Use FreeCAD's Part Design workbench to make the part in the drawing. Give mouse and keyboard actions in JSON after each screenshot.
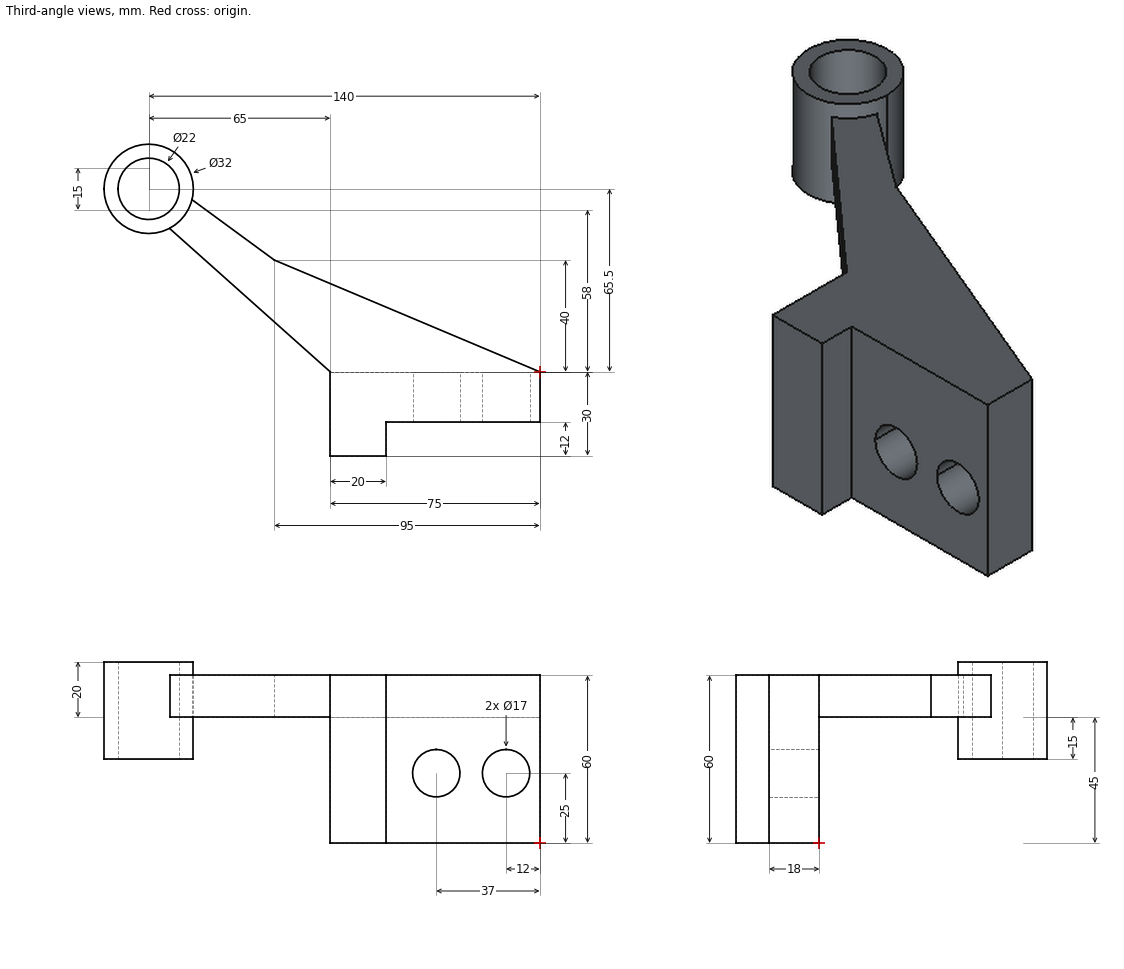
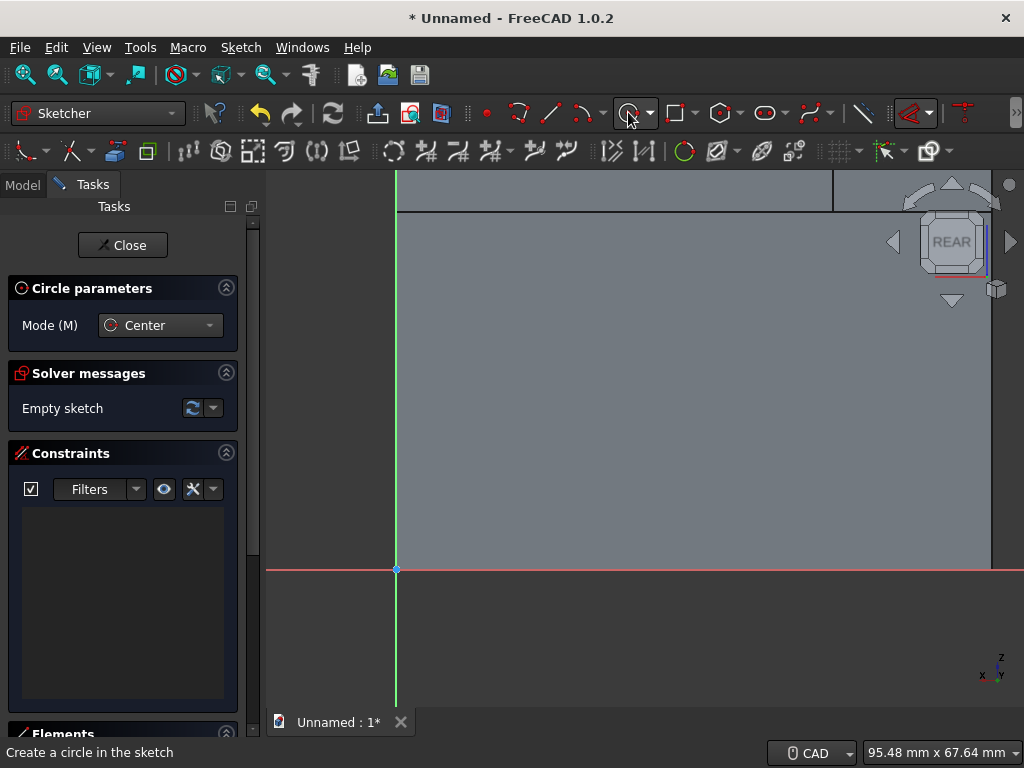
{"action": "left_click", "coordinate": [491, 371]}
{"action": "left_click", "coordinate": [539, 323]}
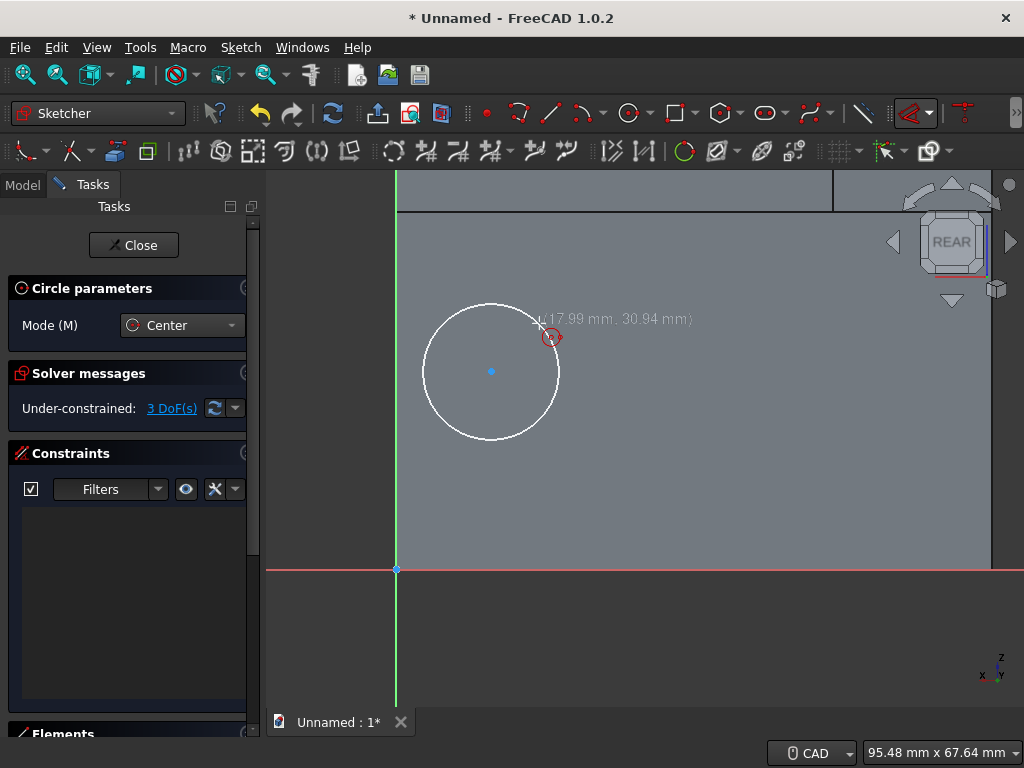
{"action": "left_click", "coordinate": [690, 371]}
{"action": "left_click", "coordinate": [738, 323]}
{"action": "key", "text": "Escape"}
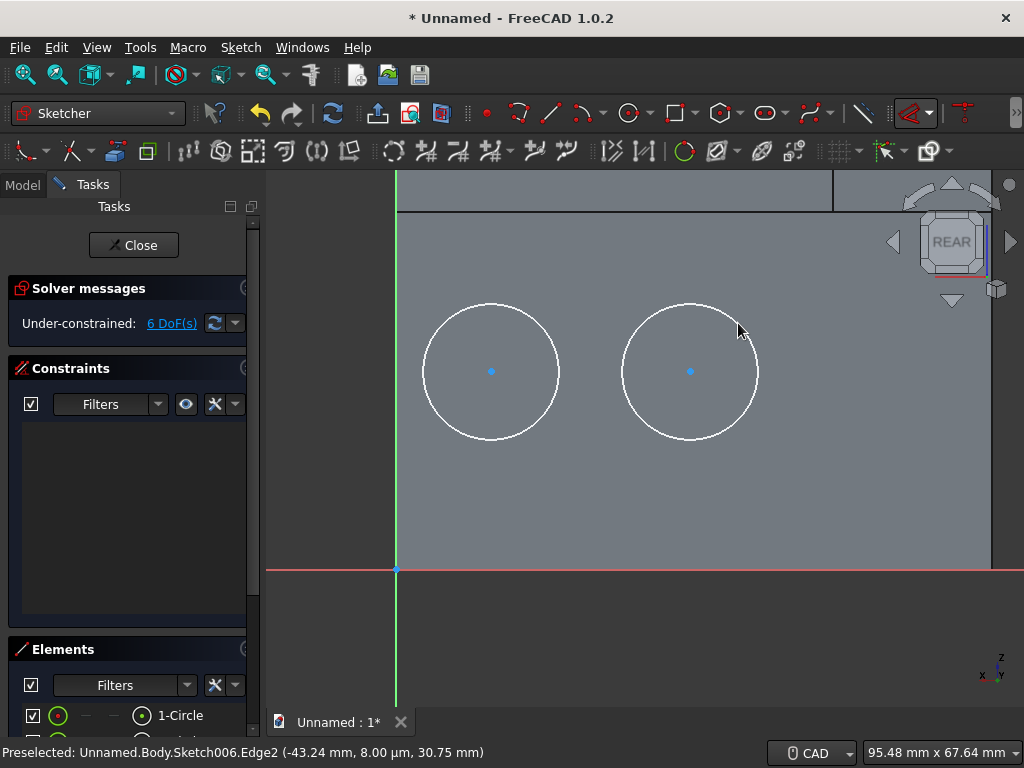
{"action": "left_click", "coordinate": [539, 324]}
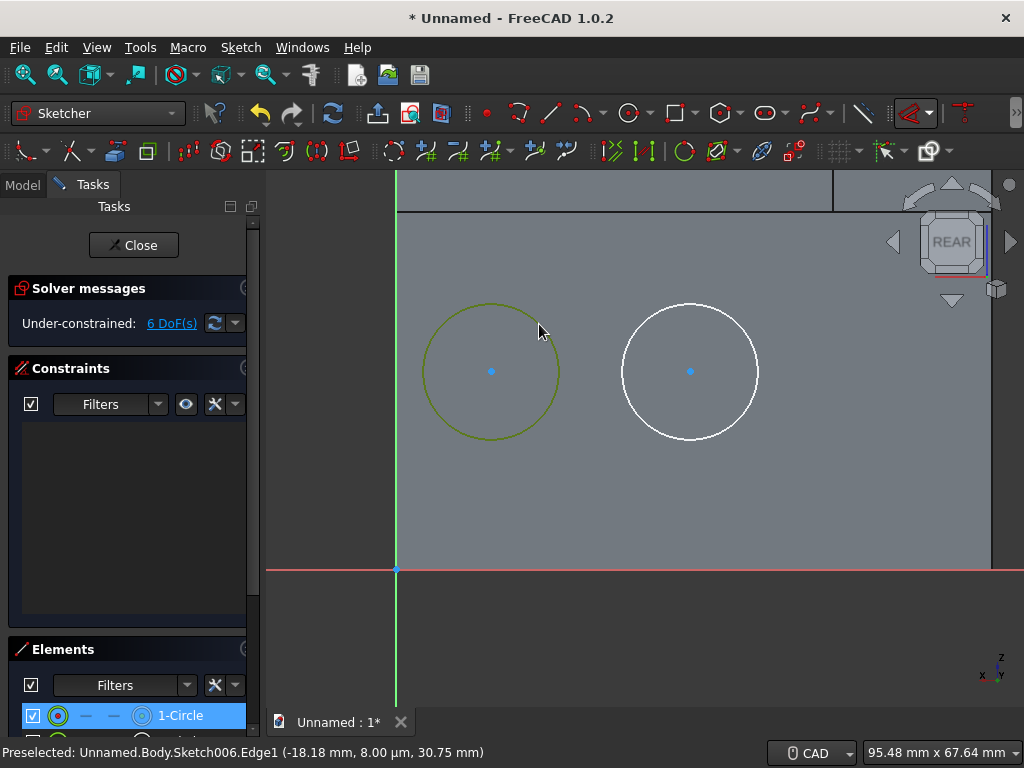
{"action": "left_click", "coordinate": [738, 324]}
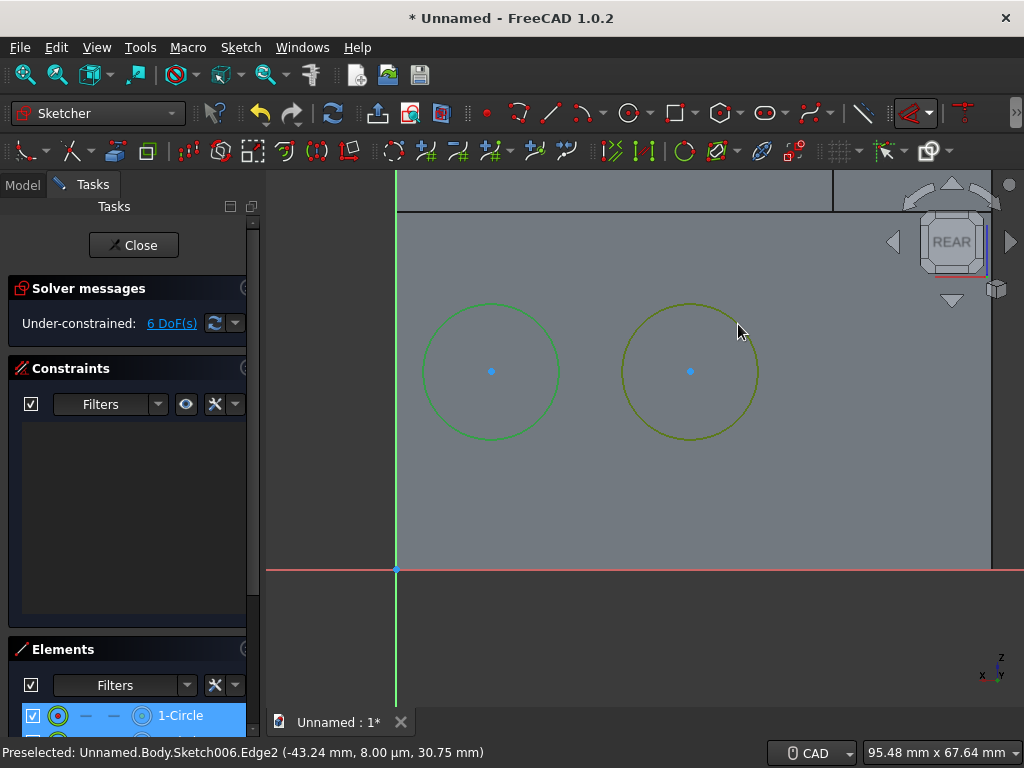
{"action": "key", "text": "e"}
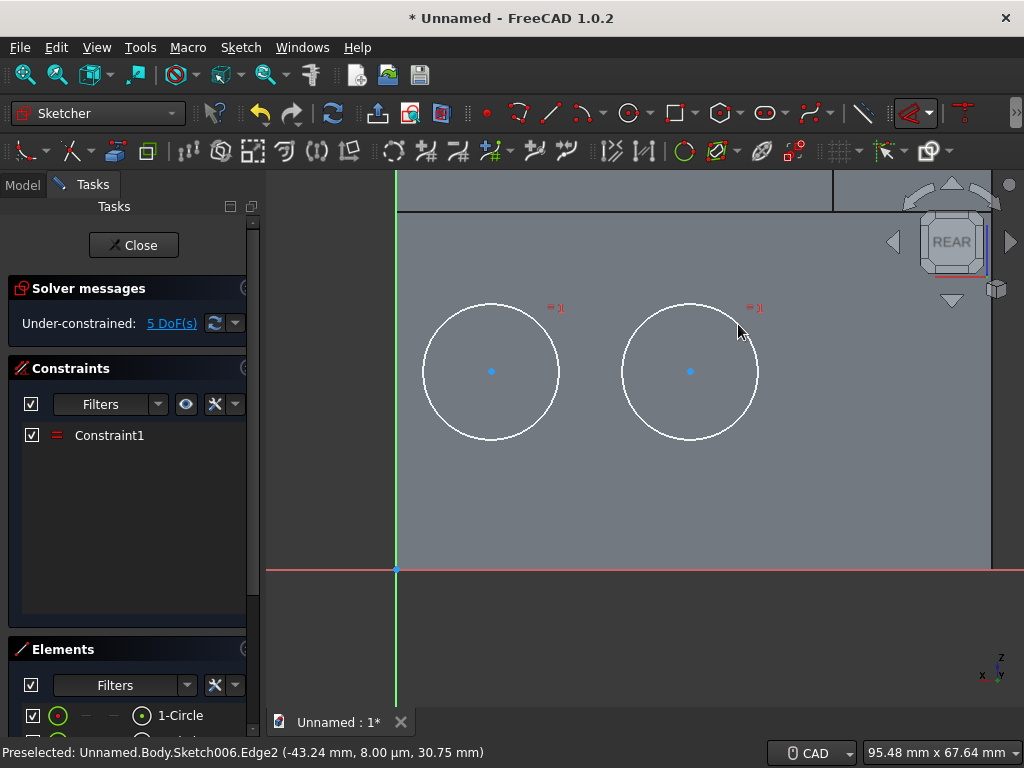
{"action": "left_click", "coordinate": [539, 324]}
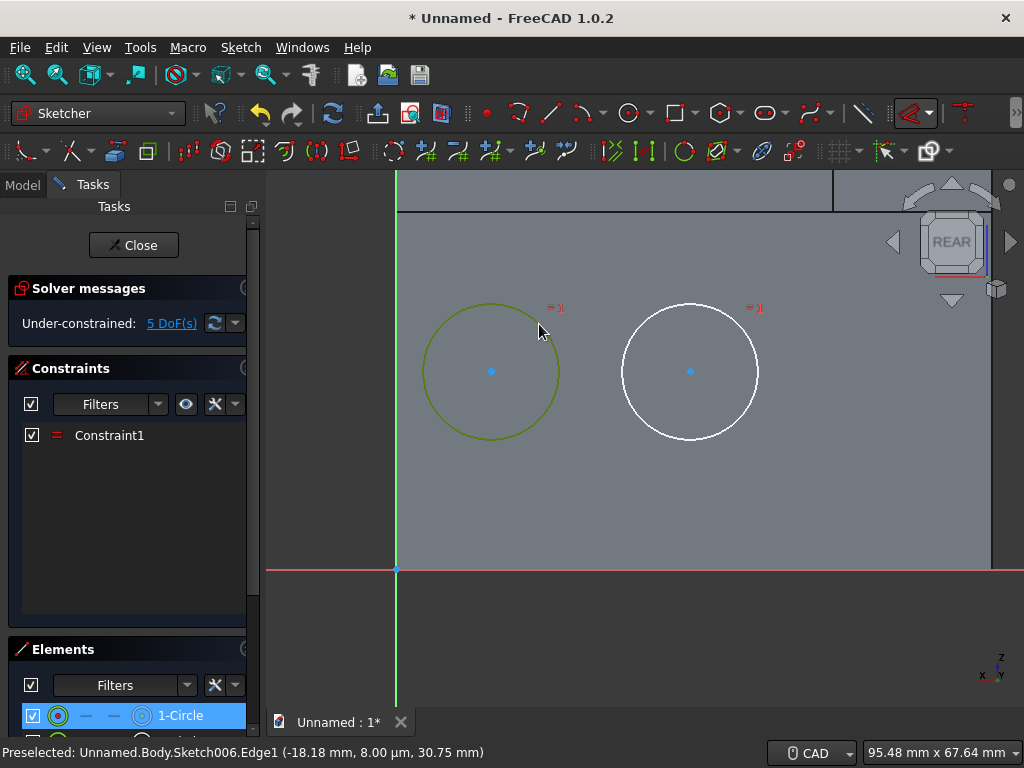
{"action": "key", "text": "k o"}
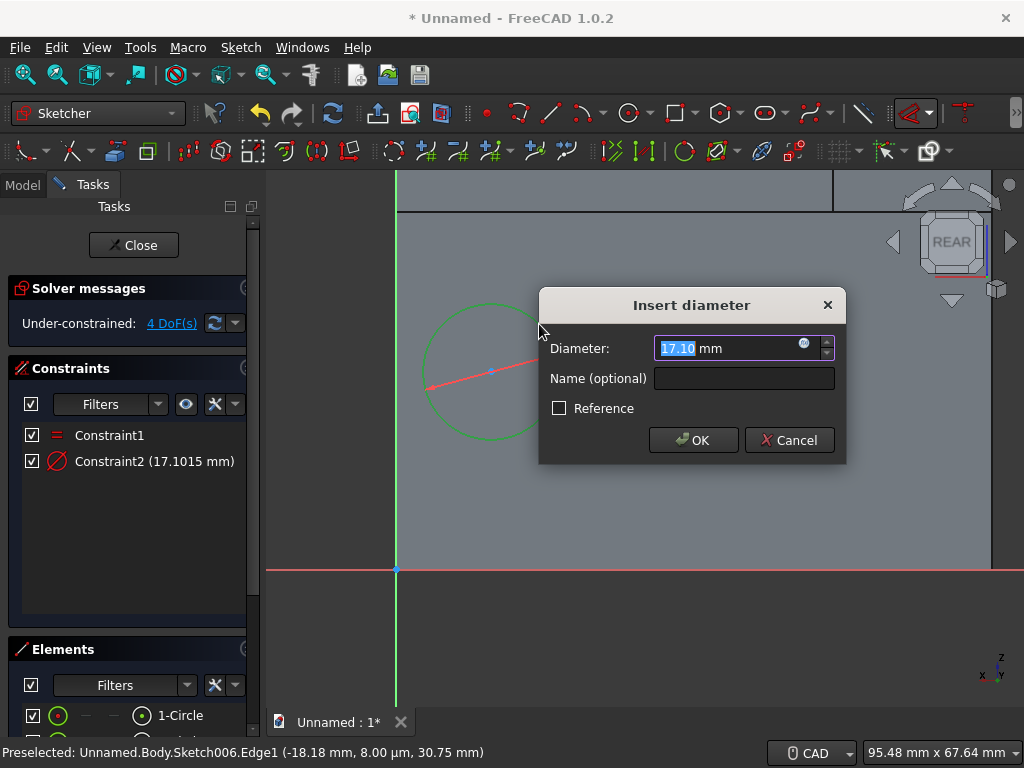
{"action": "type", "text": "17"}
{"action": "key", "text": "Return"}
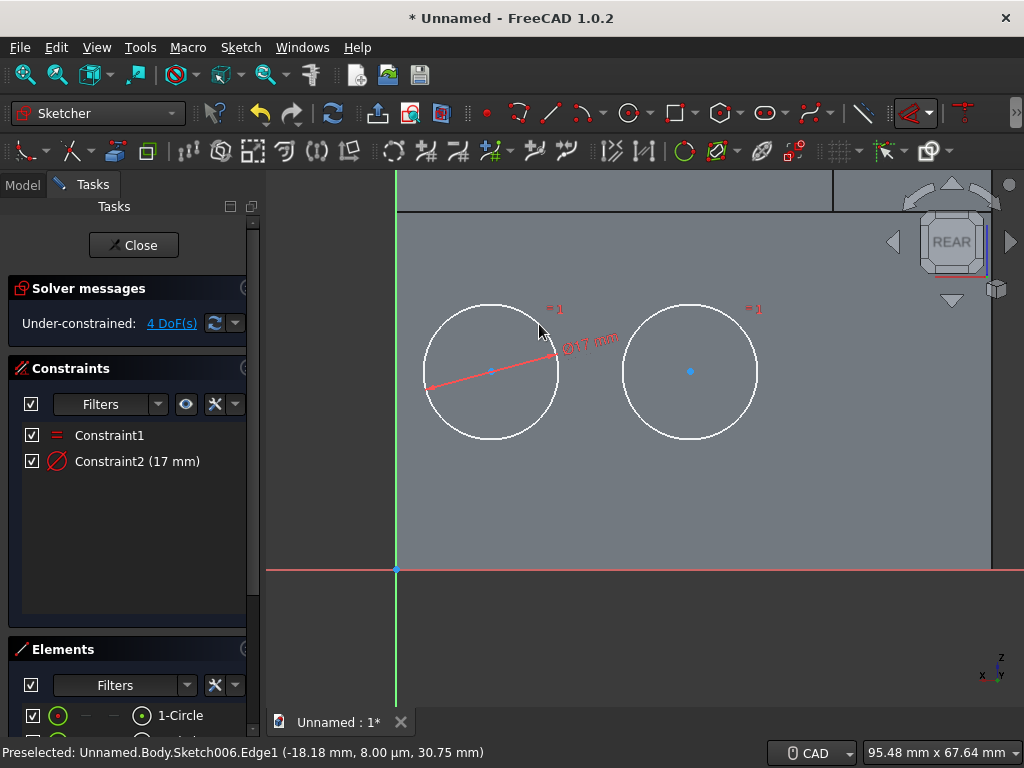
{"action": "left_click", "coordinate": [491, 372]}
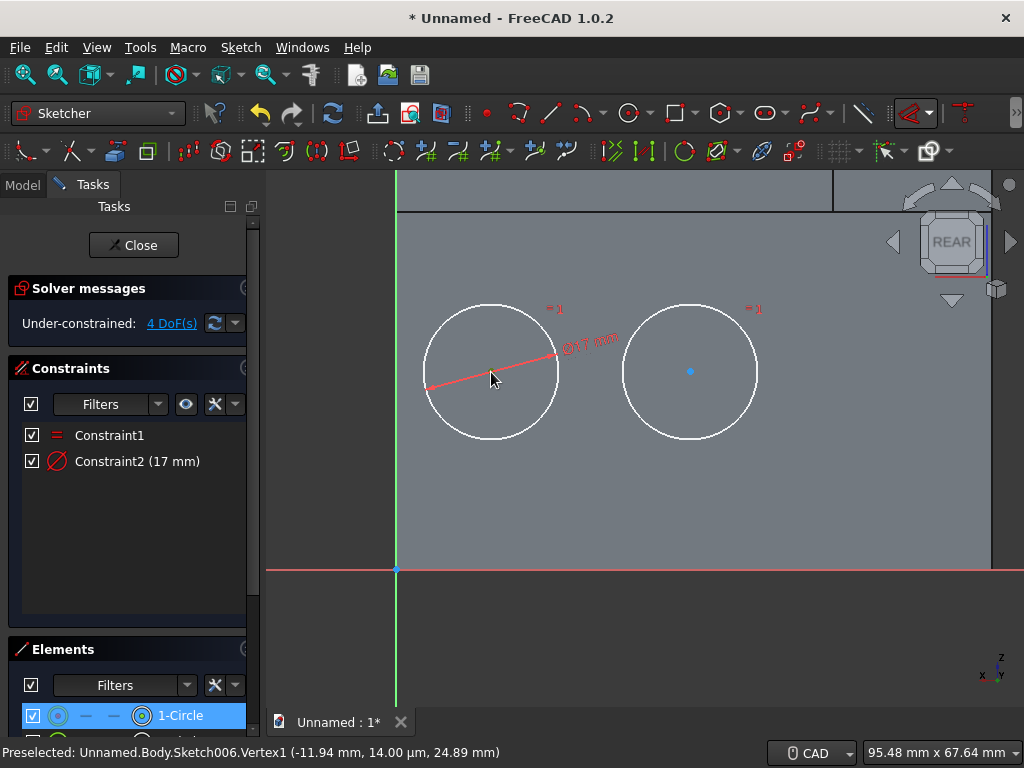
{"action": "key", "text": "l"}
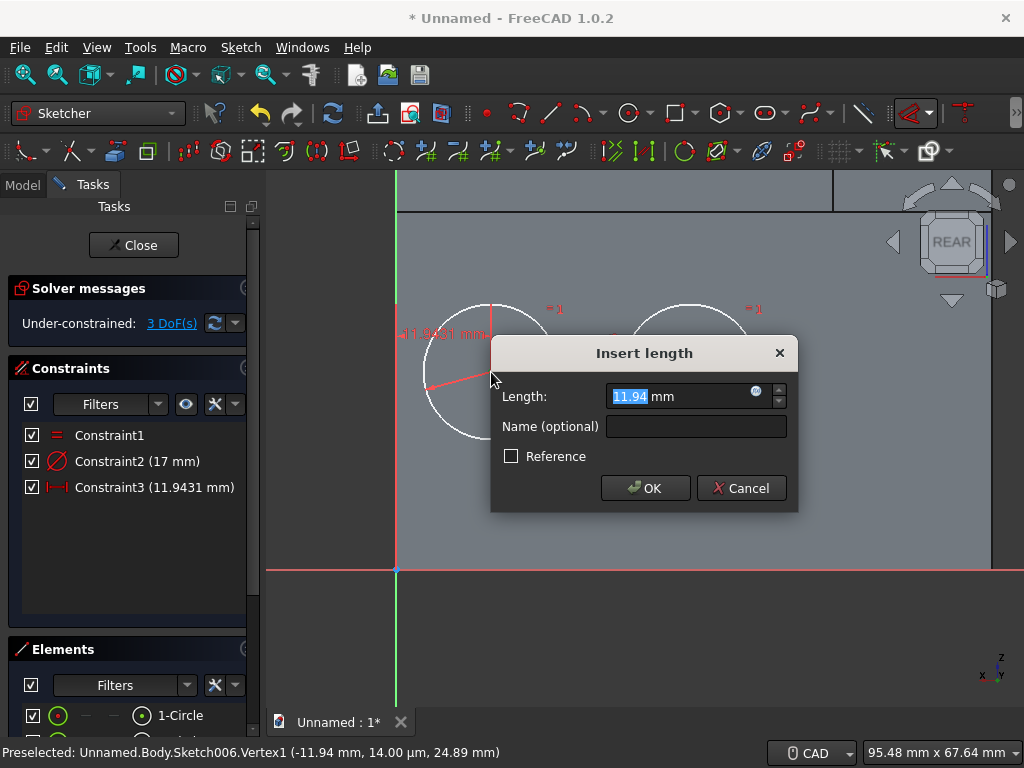
{"action": "type", "text": "12"}
{"action": "key", "text": "Return"}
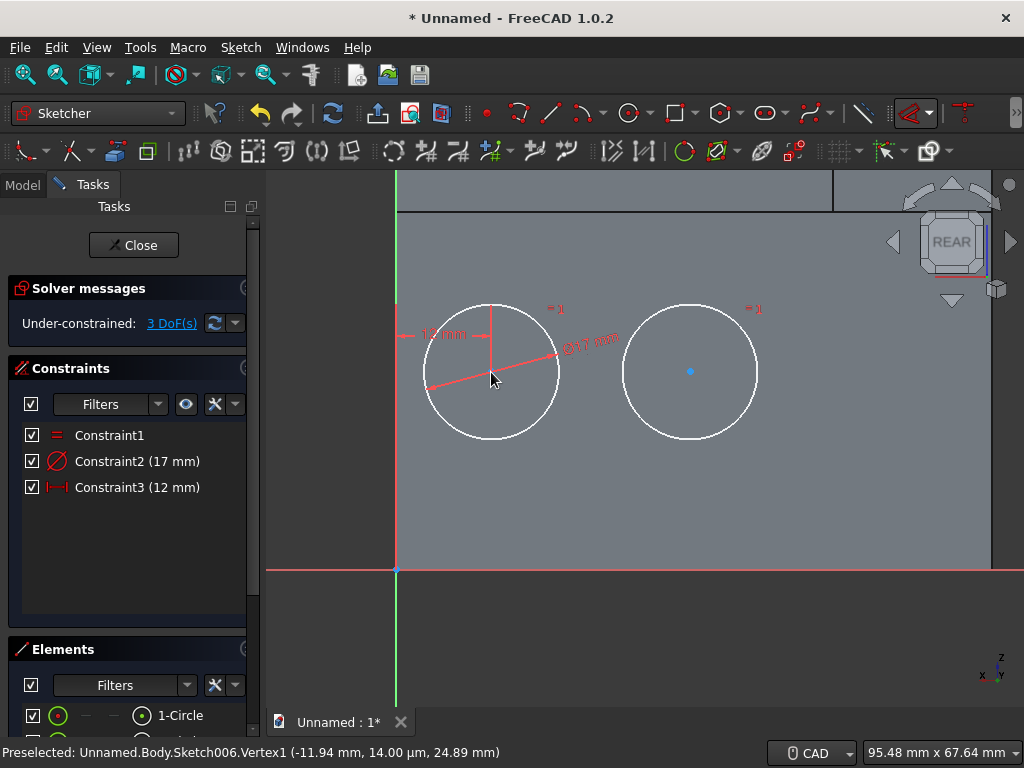
{"action": "left_click", "coordinate": [491, 372]}